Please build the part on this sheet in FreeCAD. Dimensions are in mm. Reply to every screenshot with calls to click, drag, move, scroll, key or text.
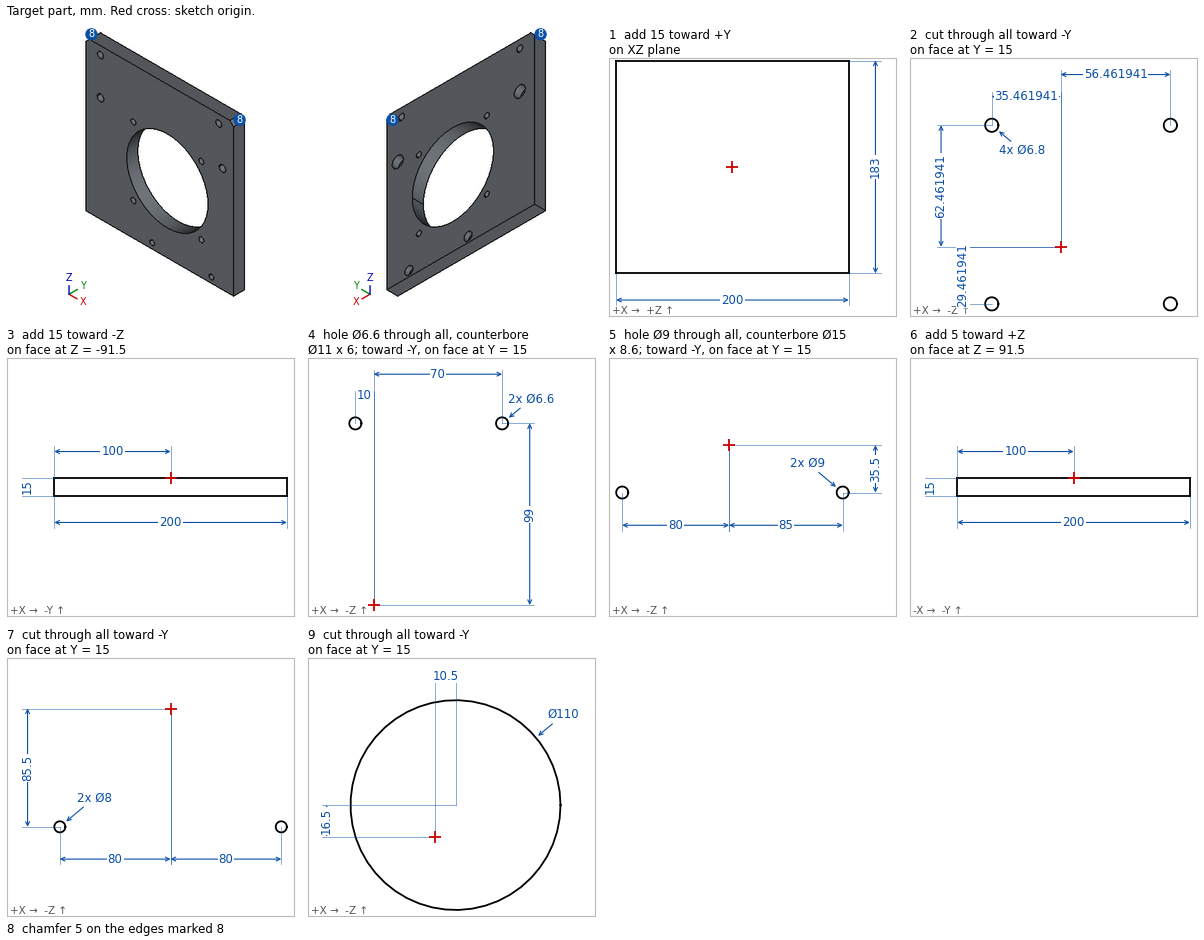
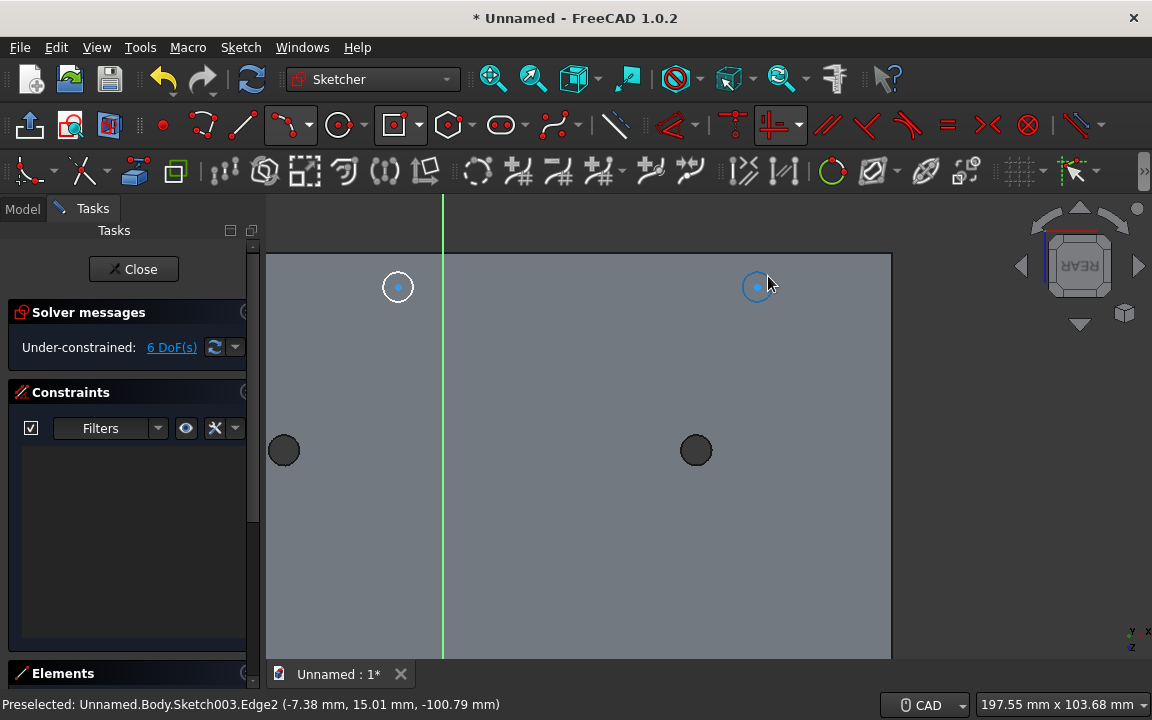
click(768, 277)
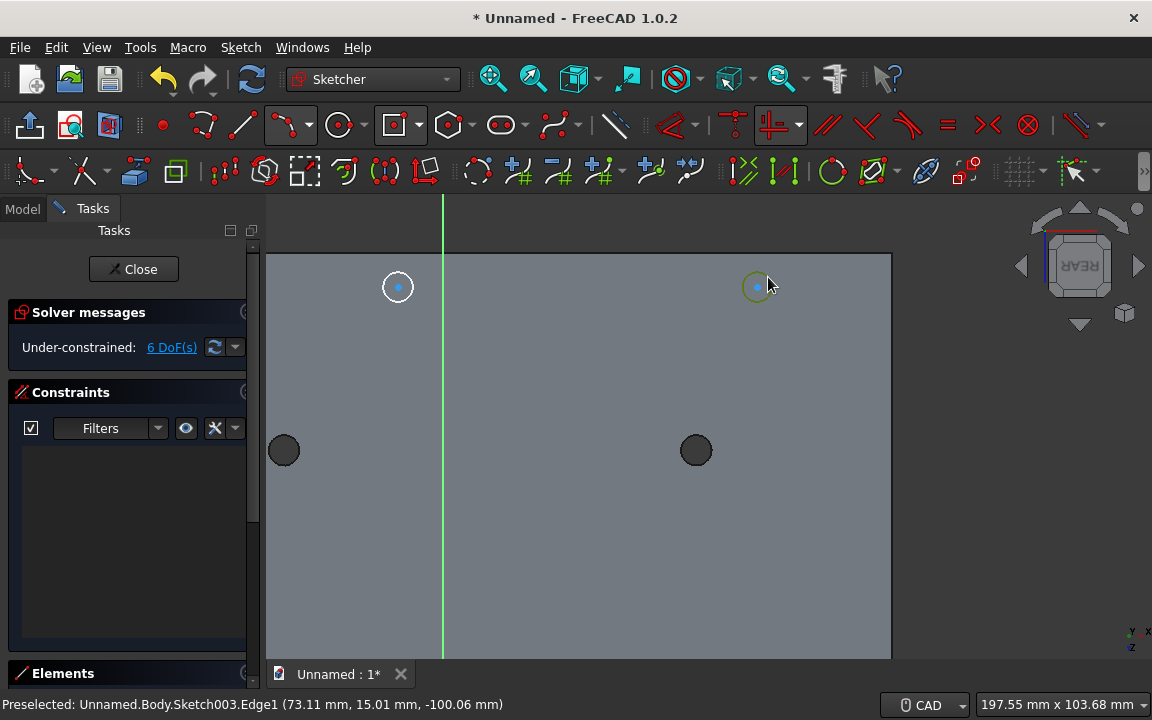
click(408, 277)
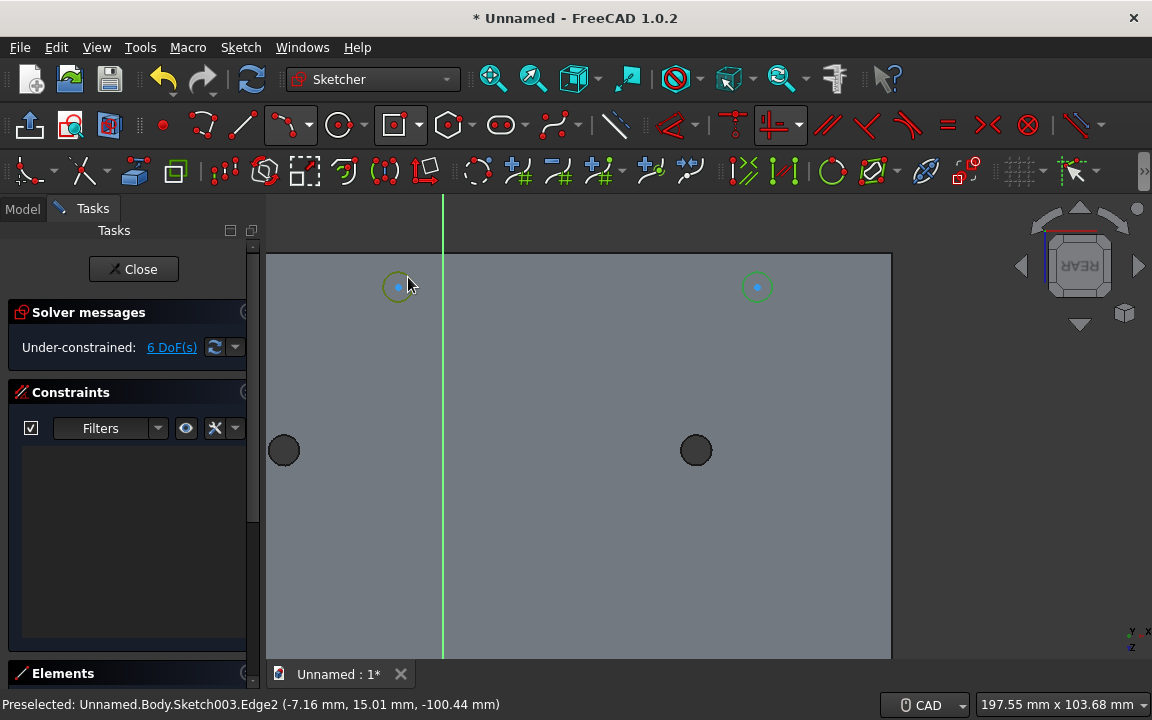
click(948, 126)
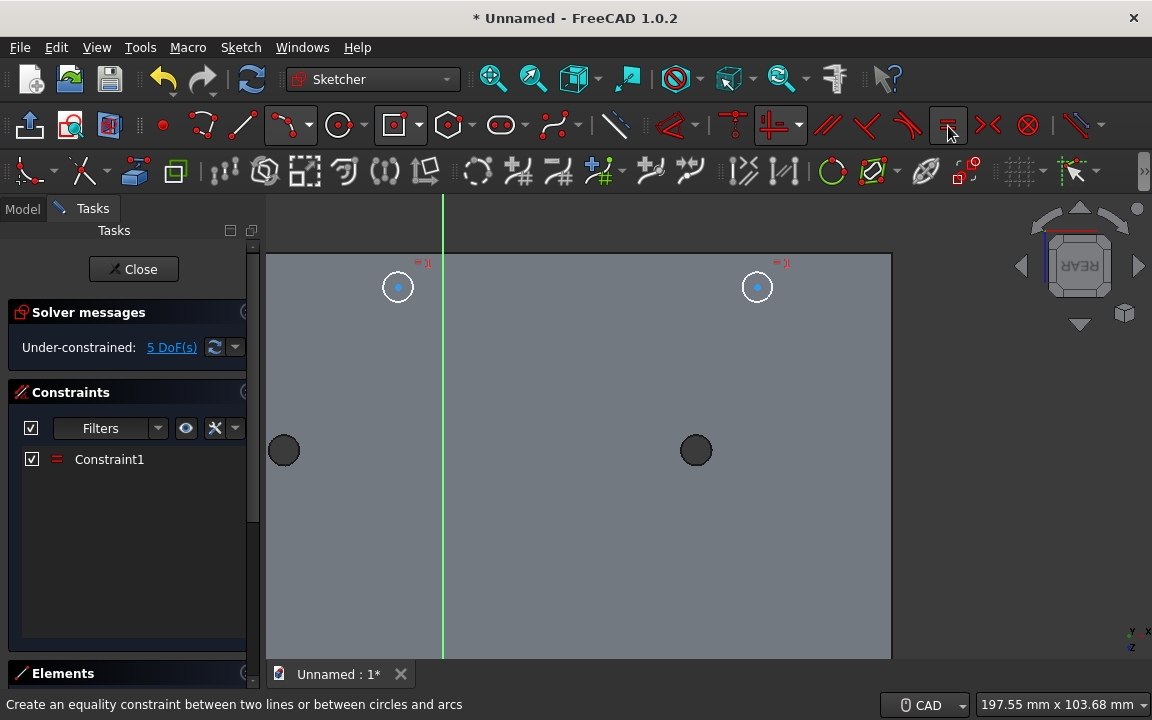
click(757, 287)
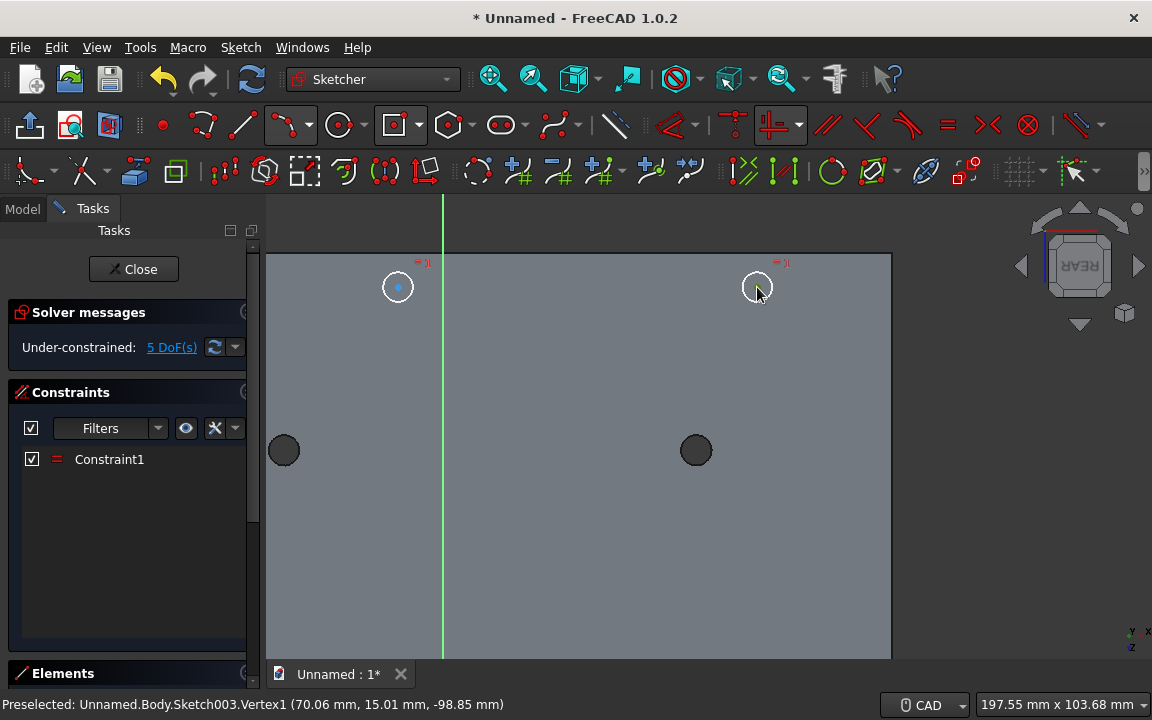
click(398, 287)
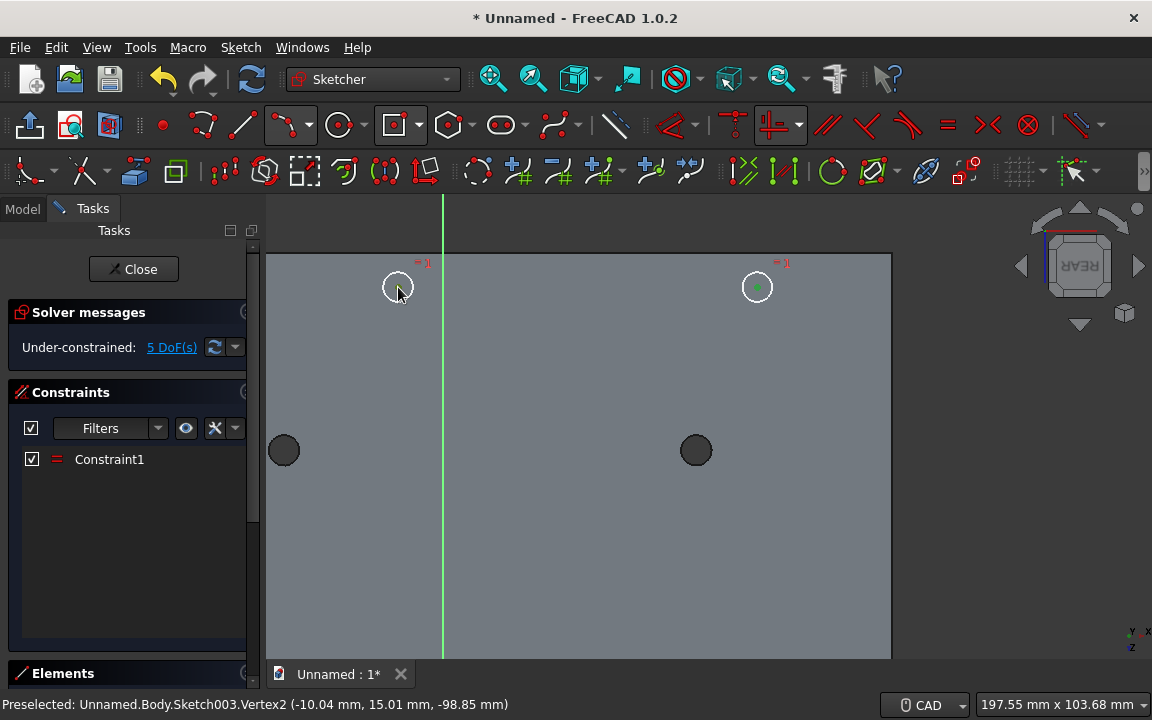
click(802, 126)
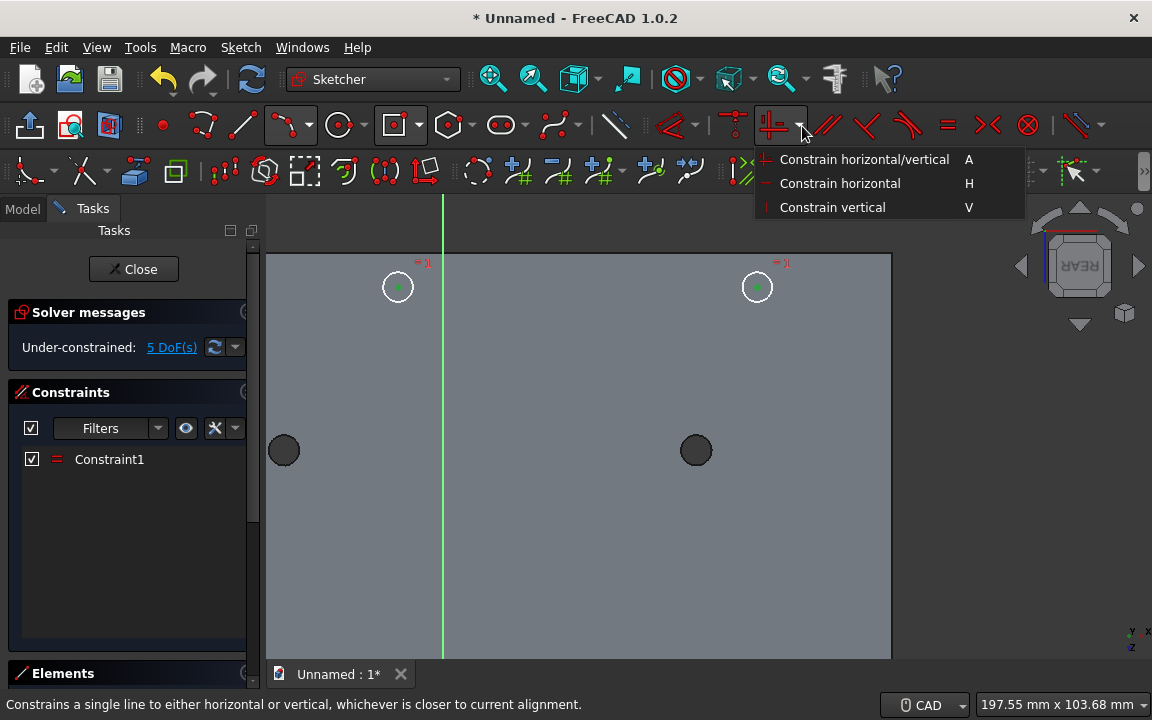
click(890, 183)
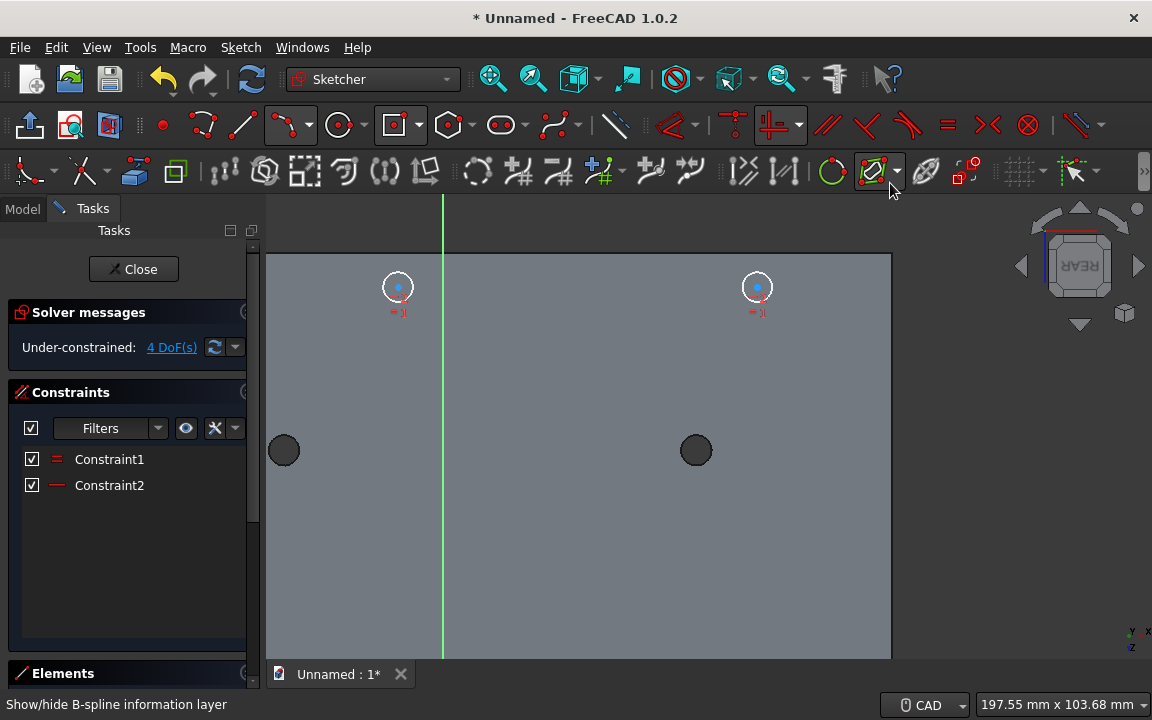
click(670, 126)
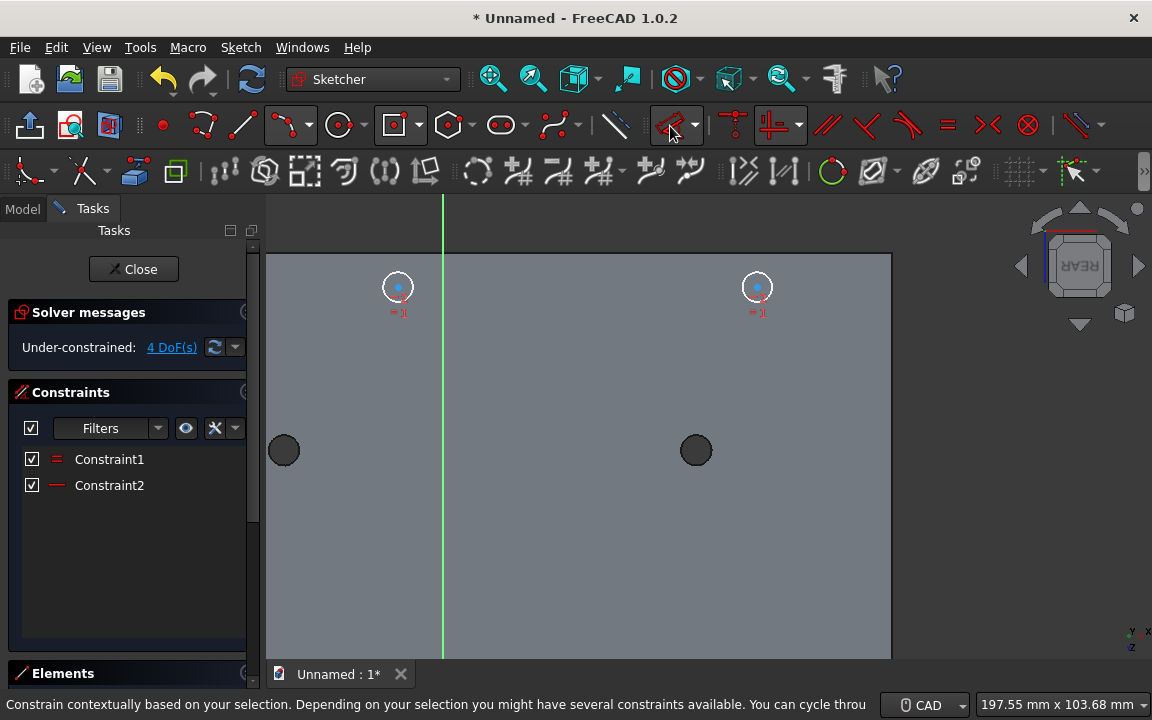
scroll(768, 277, up, 2)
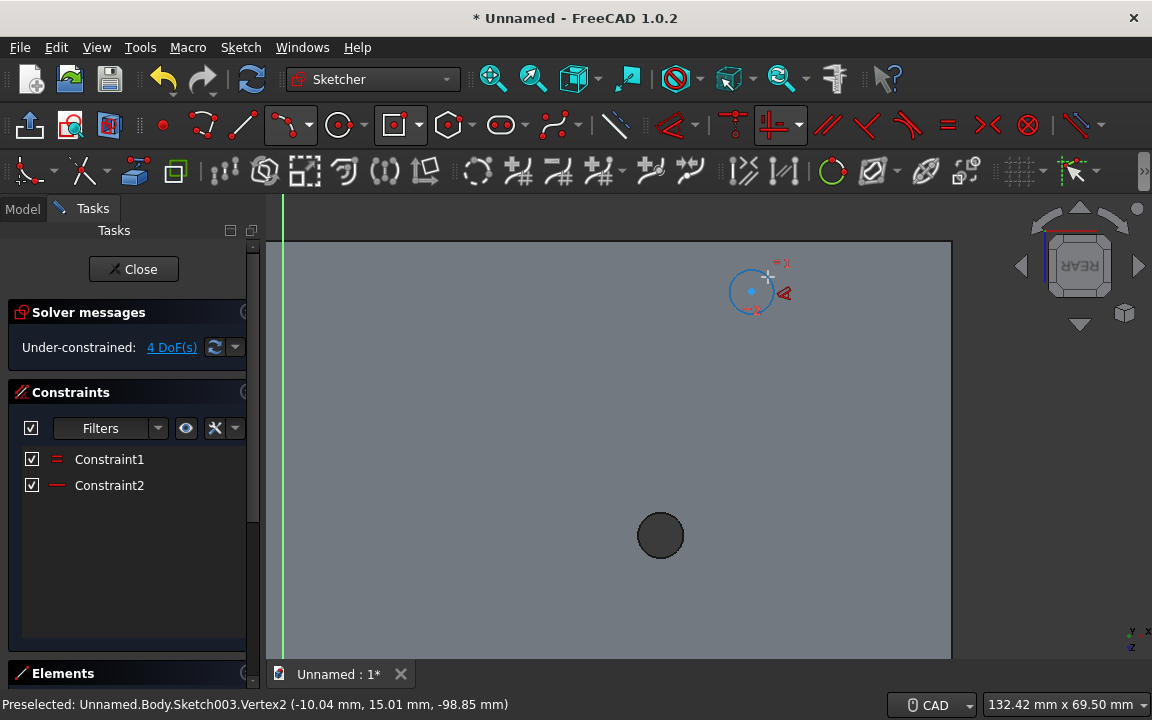
click(767, 276)
click(789, 253)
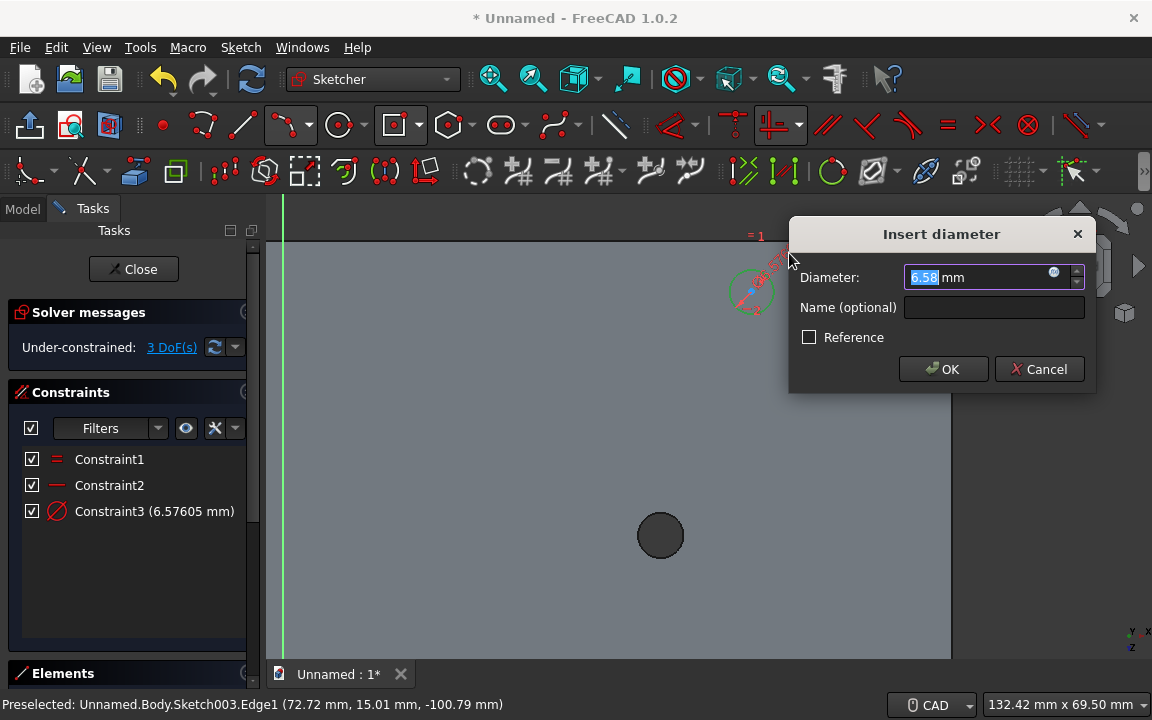
text(6.6)
key(Return)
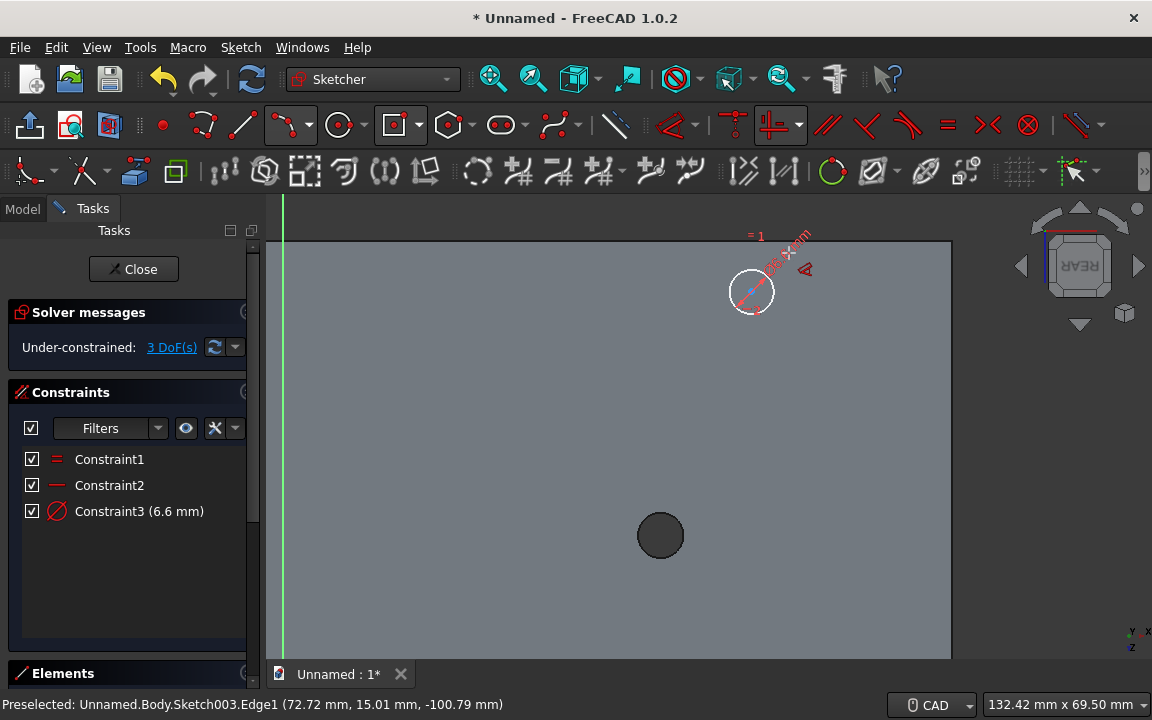
click(752, 292)
click(523, 258)